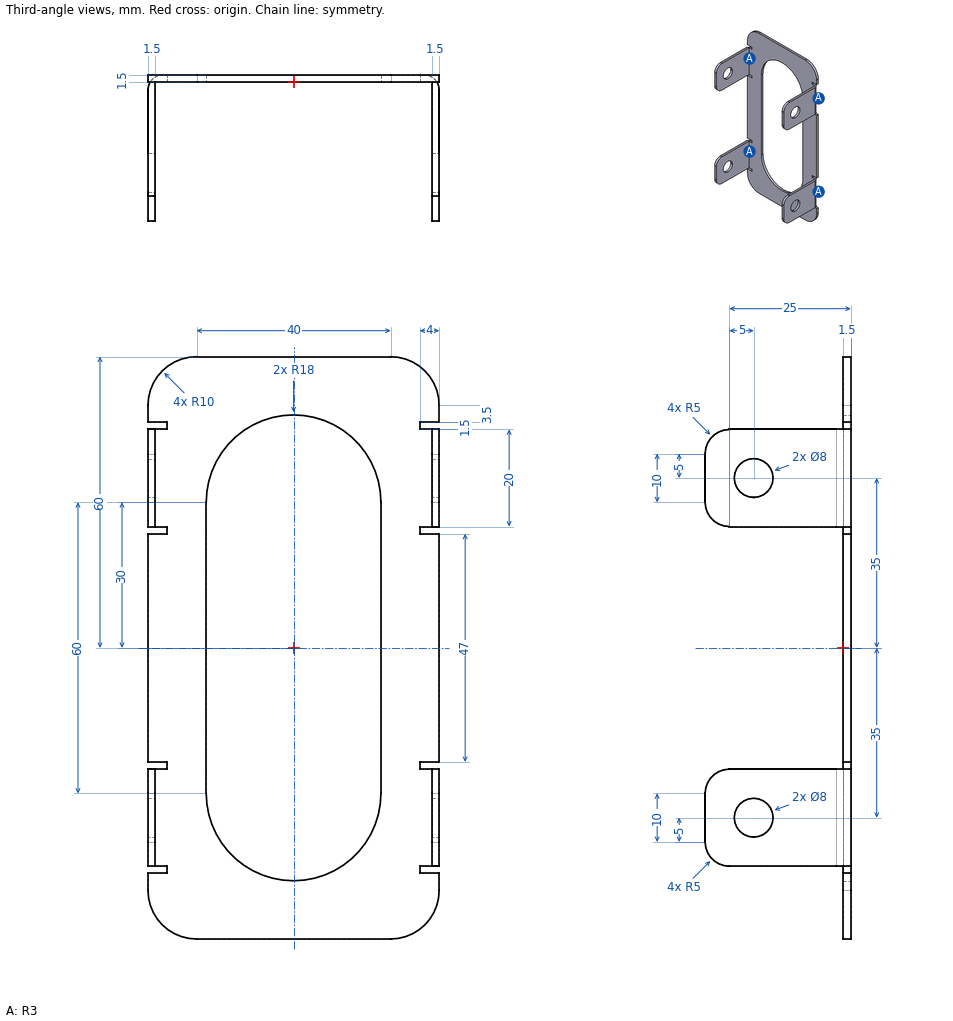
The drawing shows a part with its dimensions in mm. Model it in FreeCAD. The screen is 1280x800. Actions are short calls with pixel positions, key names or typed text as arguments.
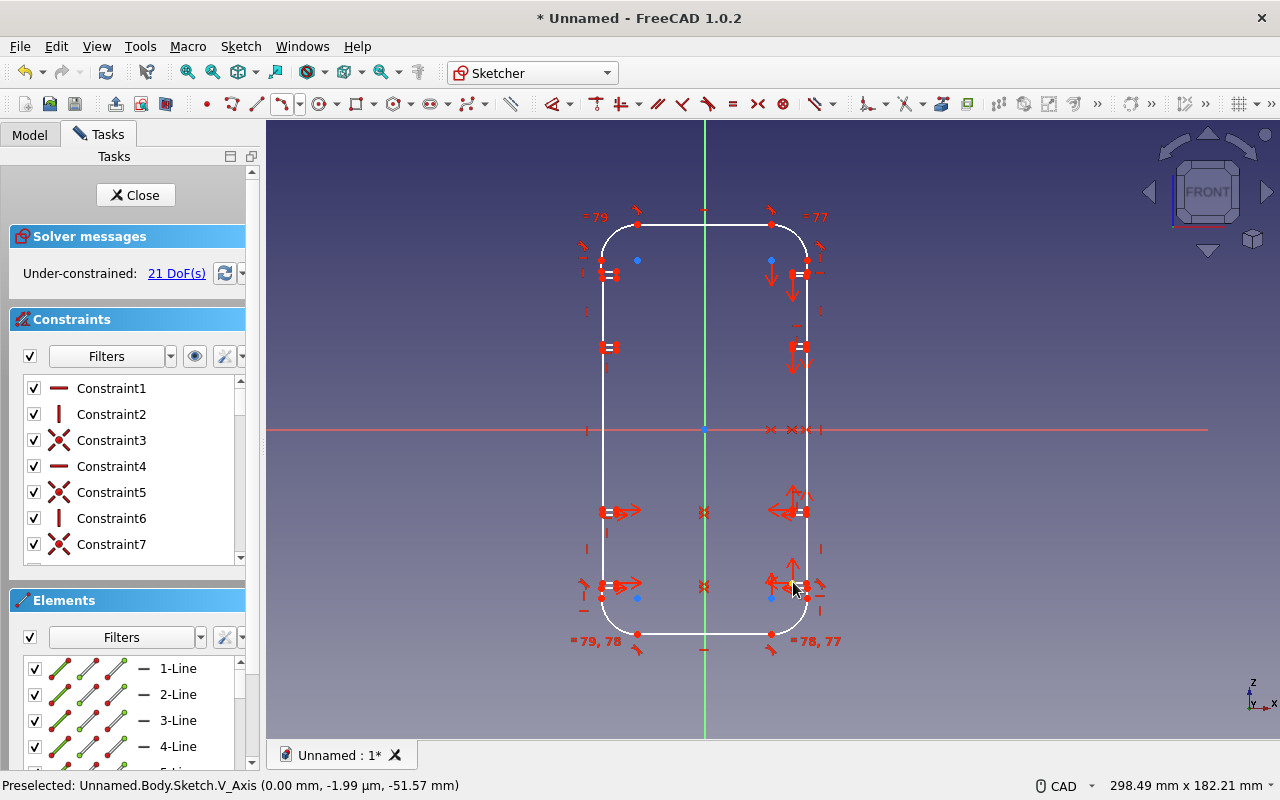
scroll(807, 349, up, 5)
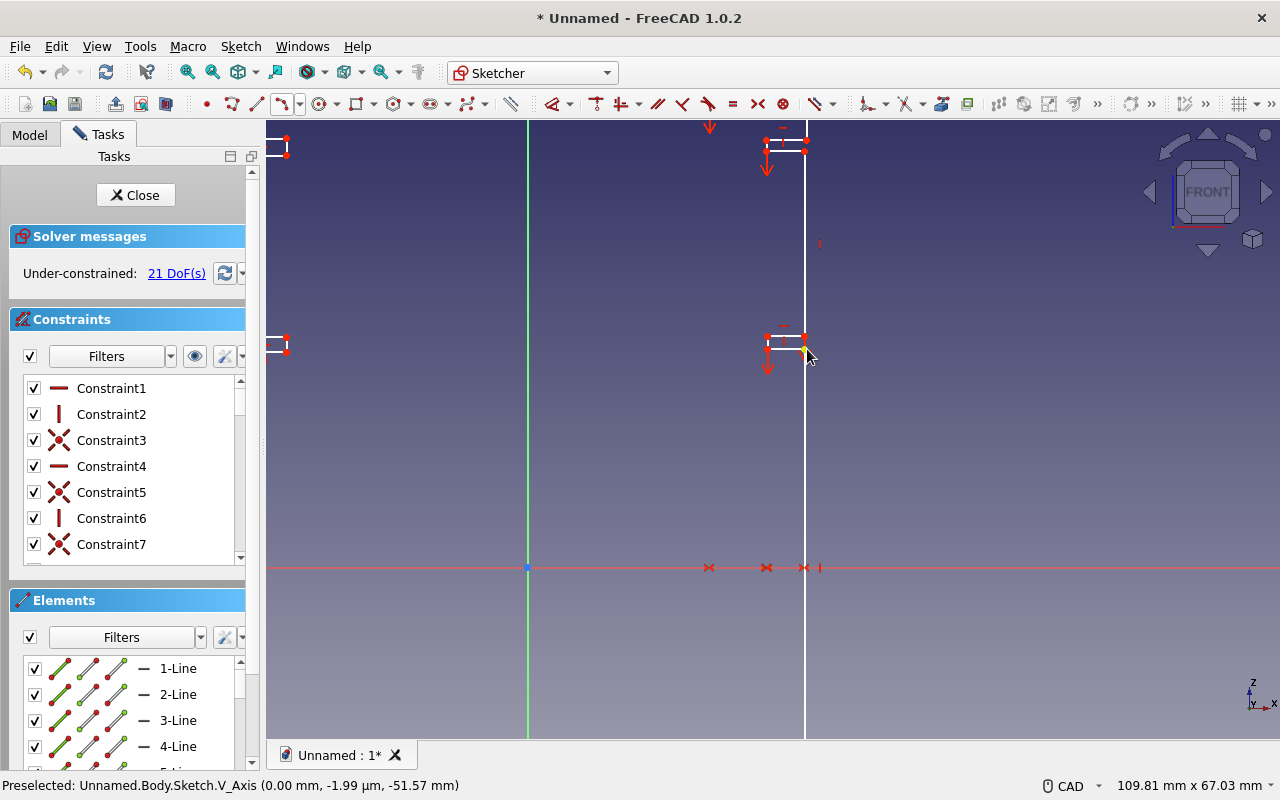
click(805, 349)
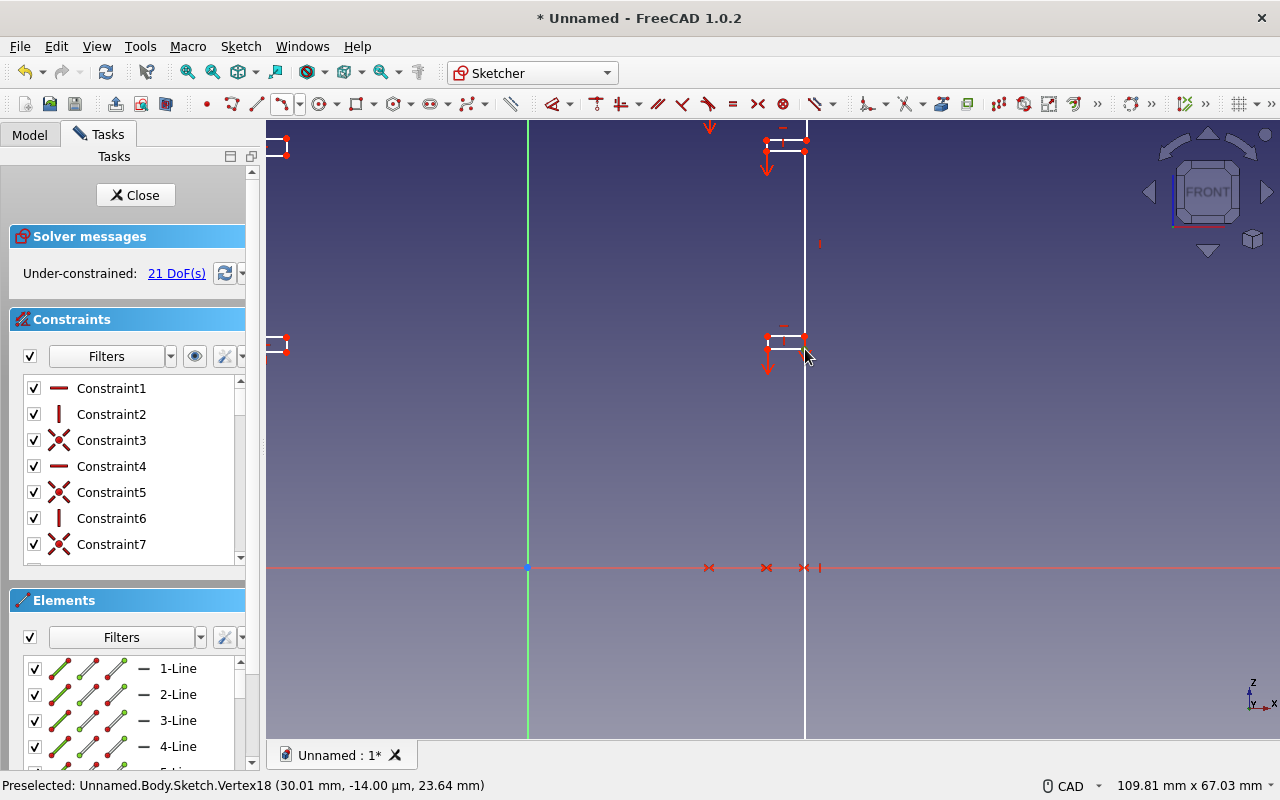
scroll(807, 349, down, 5)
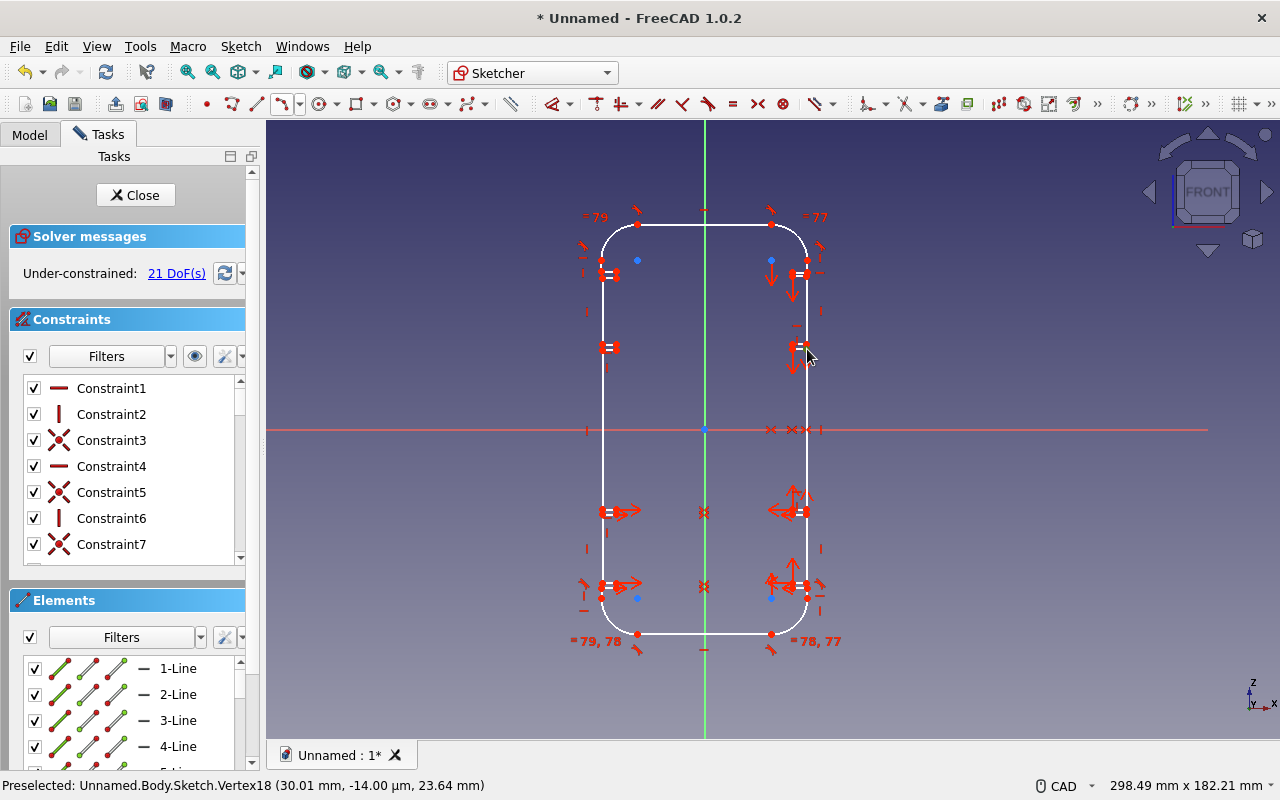
scroll(603, 350, up, 5)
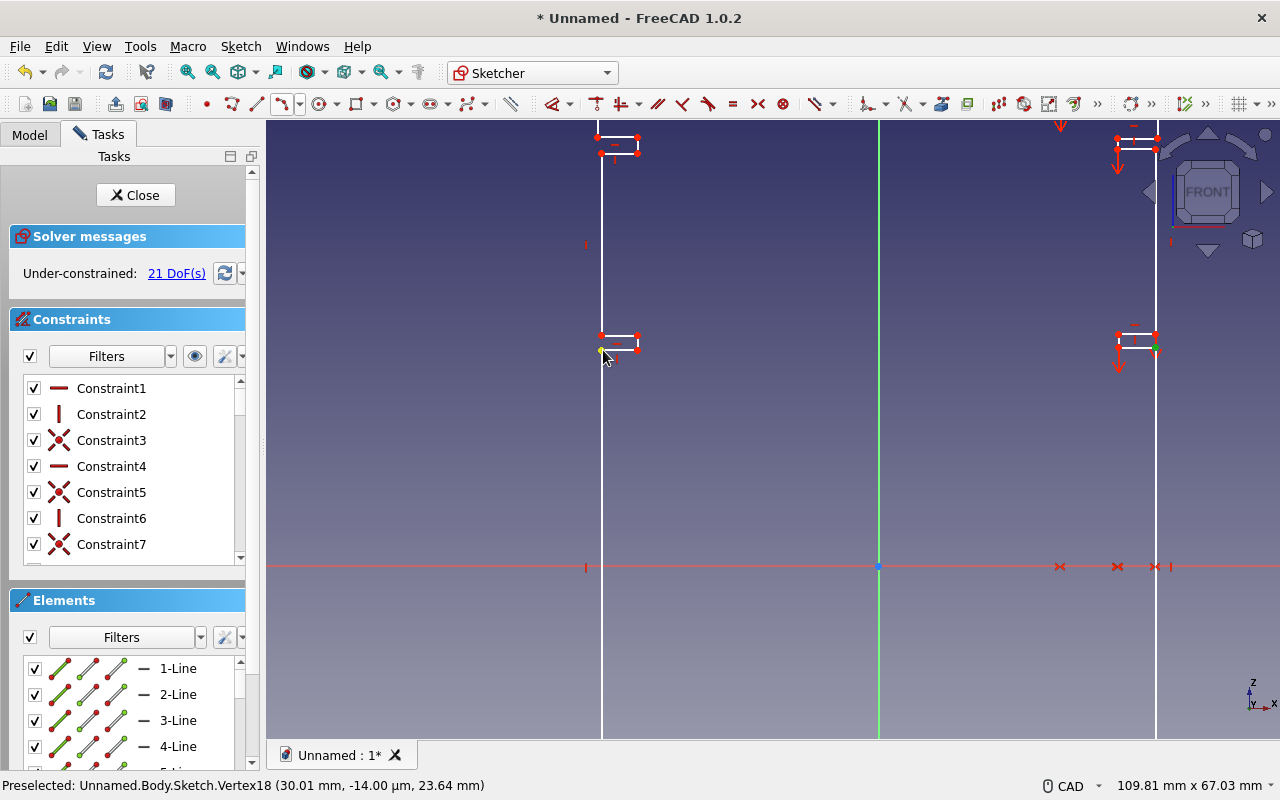
click(602, 350)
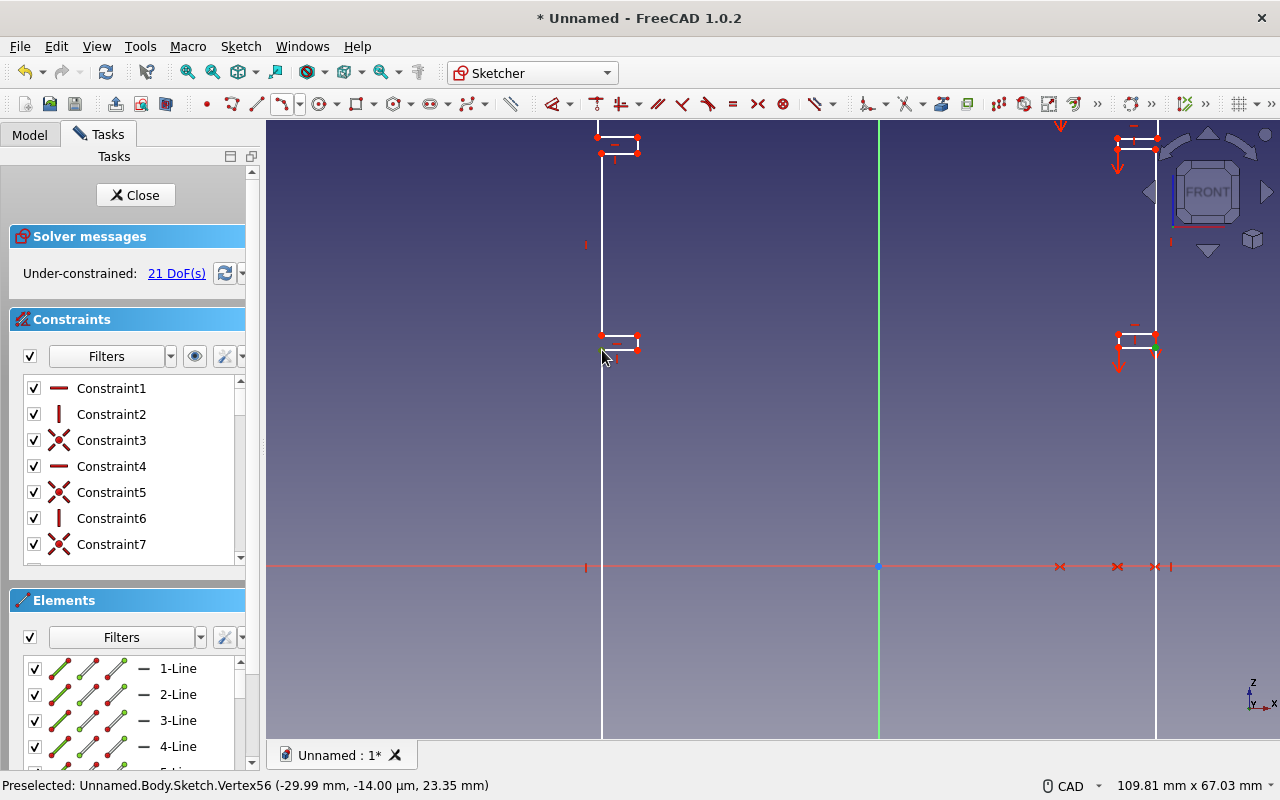
click(879, 671)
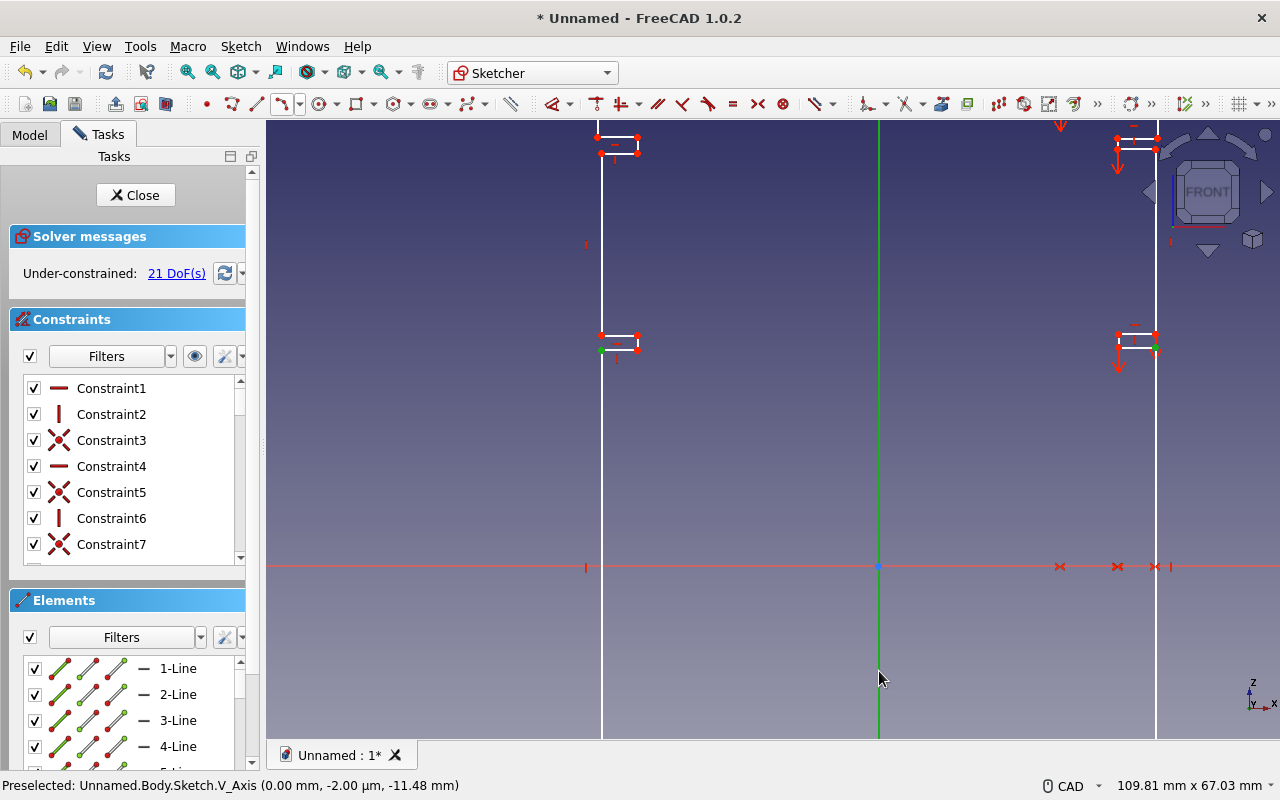
key(s)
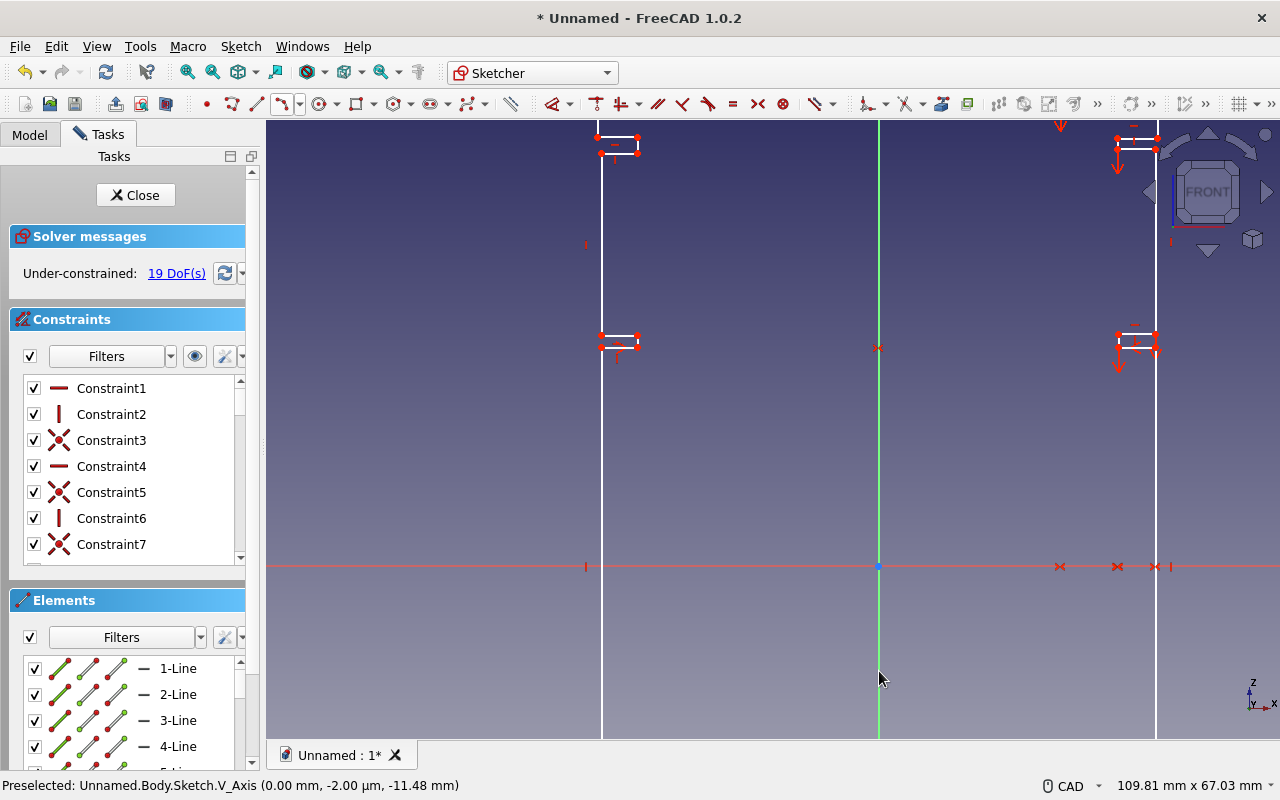
scroll(603, 350, down, 5)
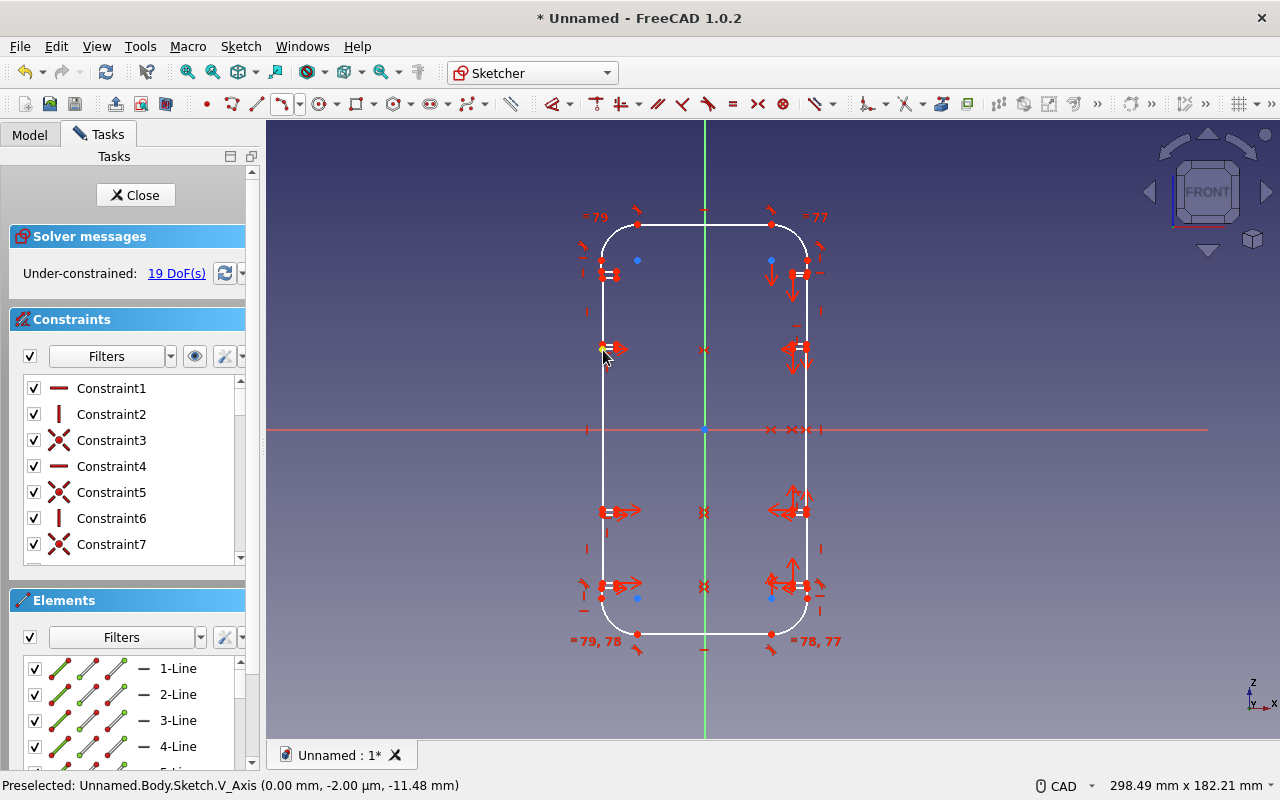
scroll(793, 344, up, 5)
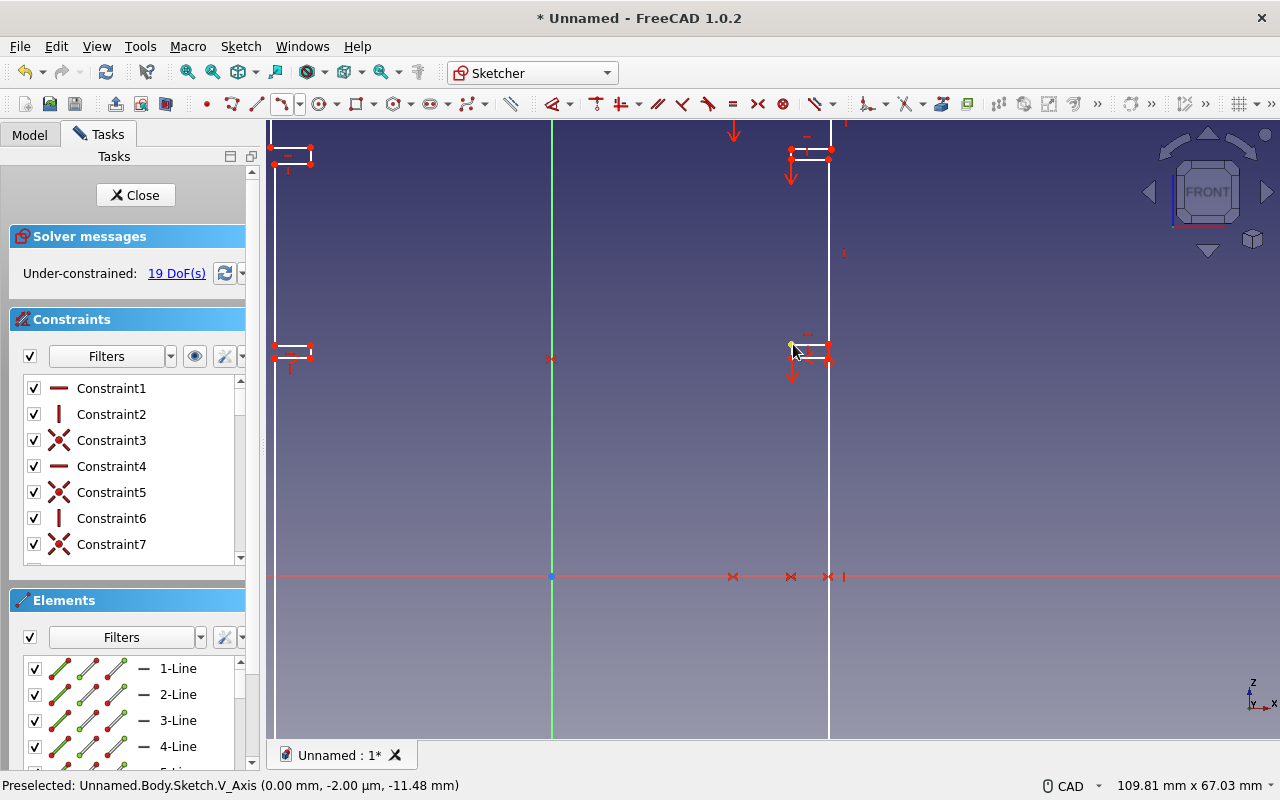
click(792, 345)